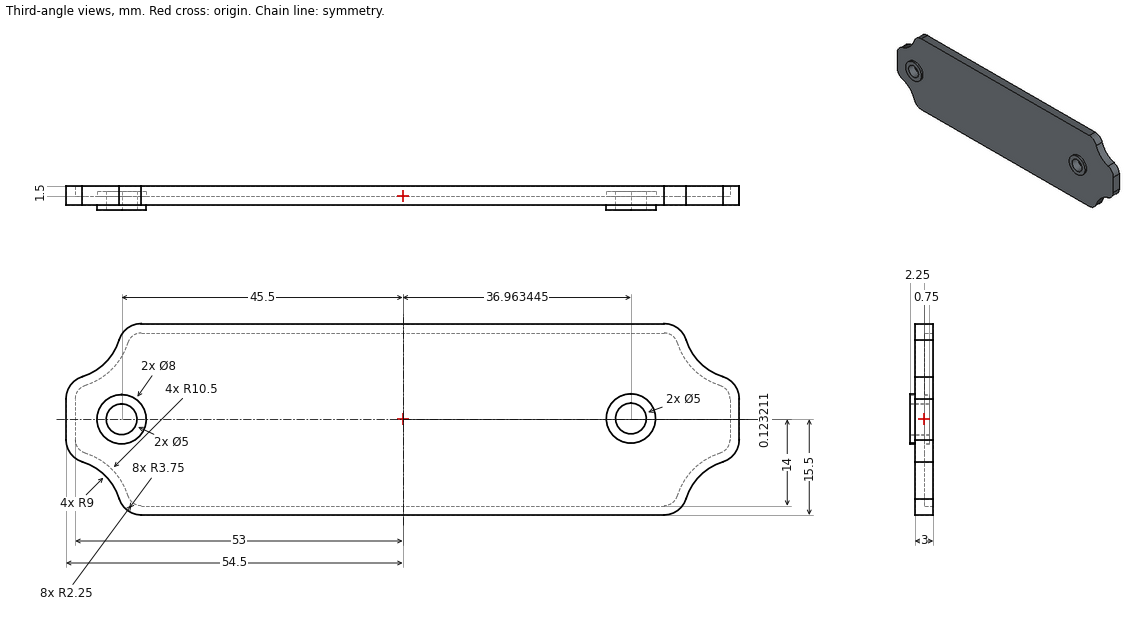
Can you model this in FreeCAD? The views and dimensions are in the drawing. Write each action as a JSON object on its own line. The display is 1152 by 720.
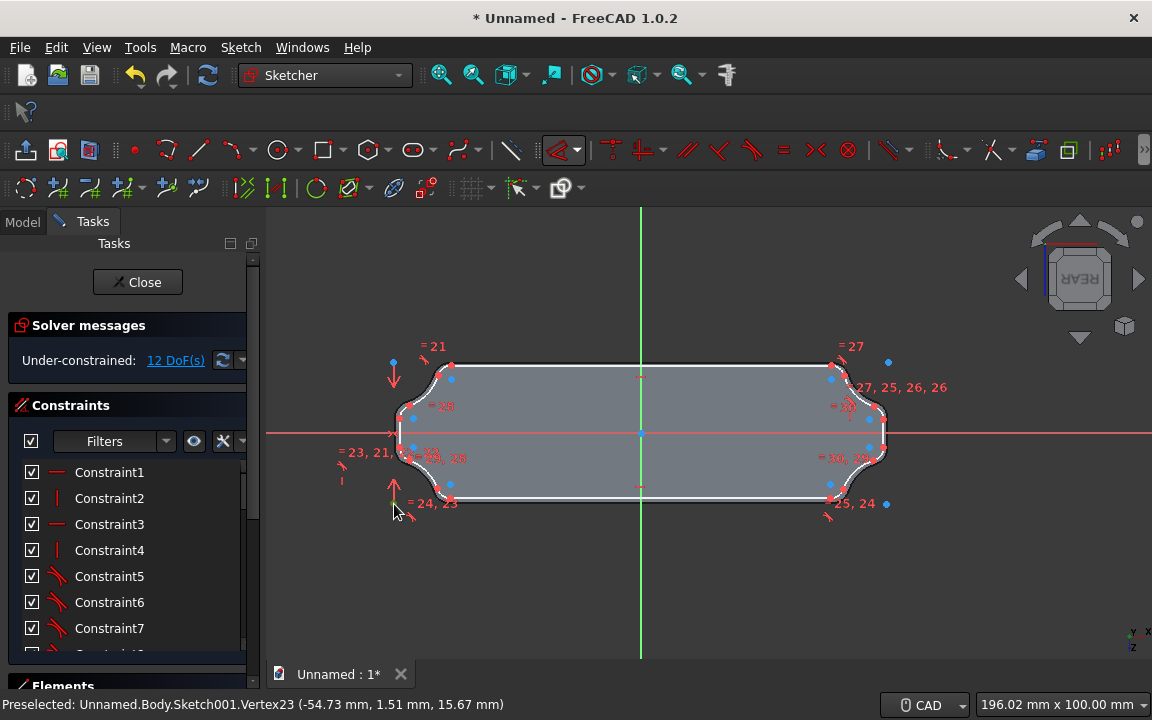
{"action": "left_click", "coordinate": [887, 505]}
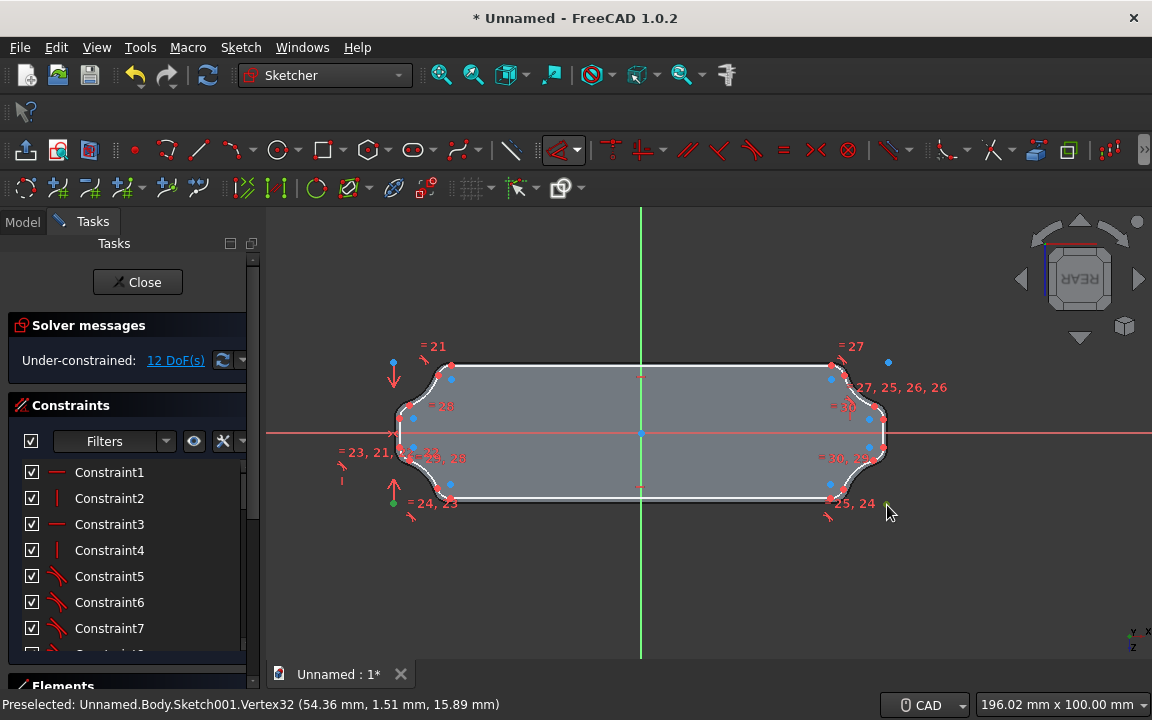
{"action": "left_click", "coordinate": [641, 603]}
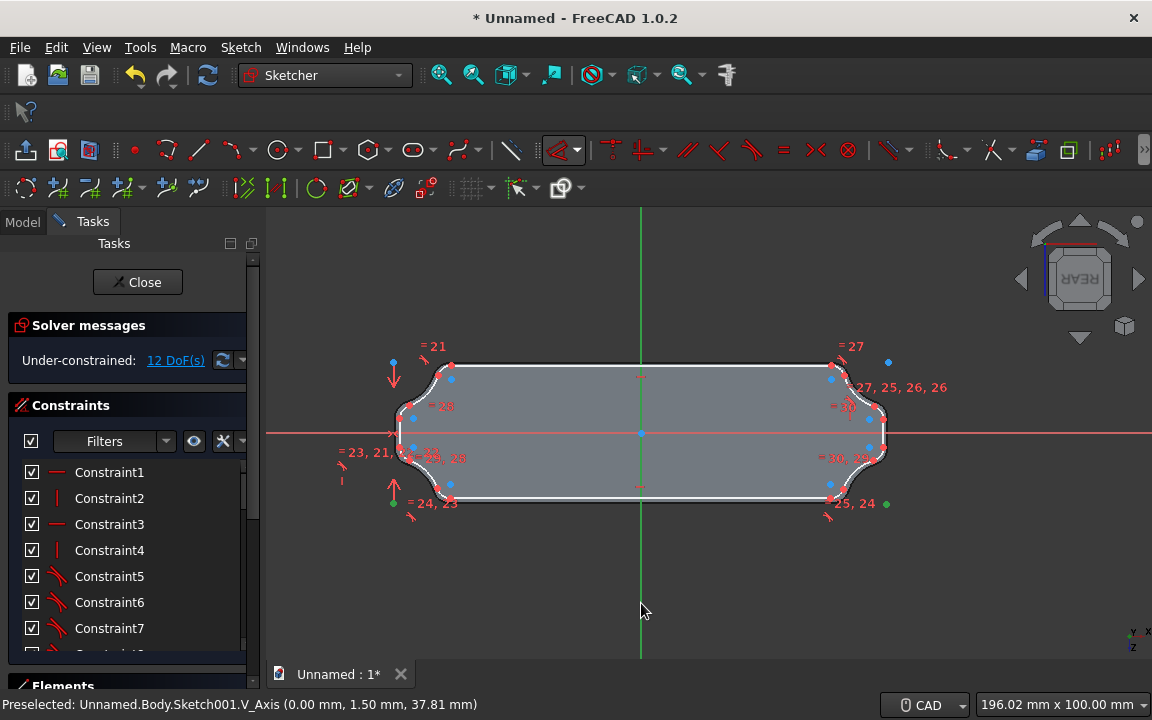
{"action": "left_click", "coordinate": [816, 150]}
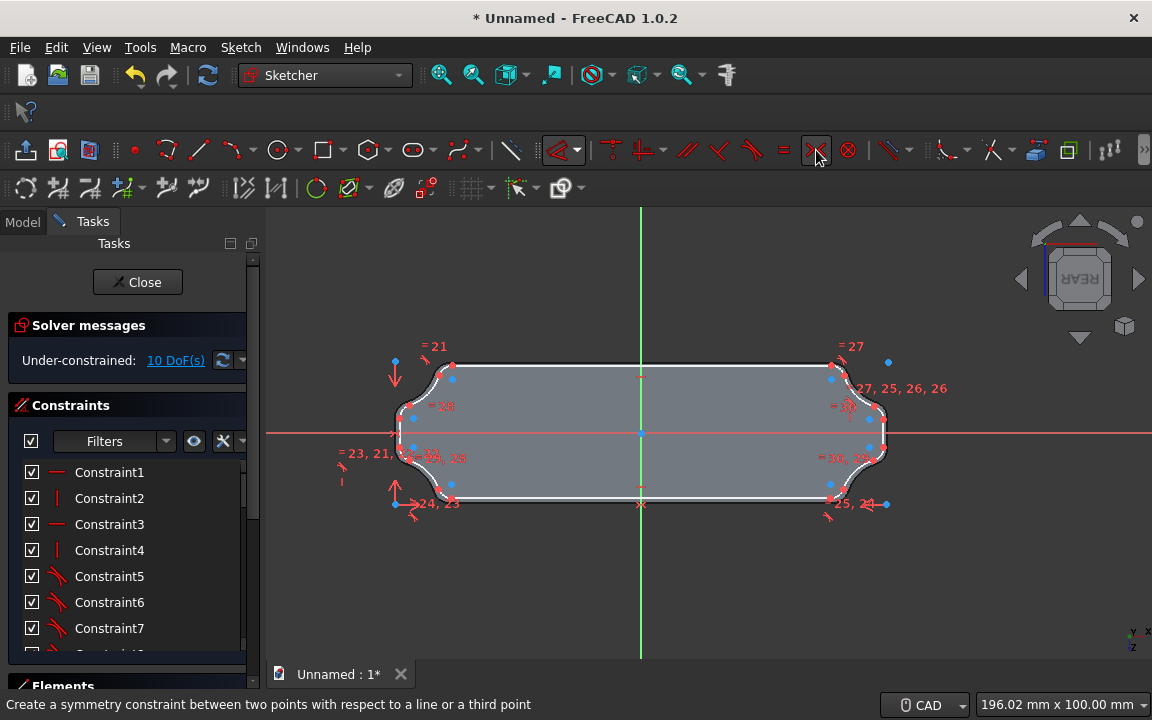
{"action": "left_click", "coordinate": [414, 418]}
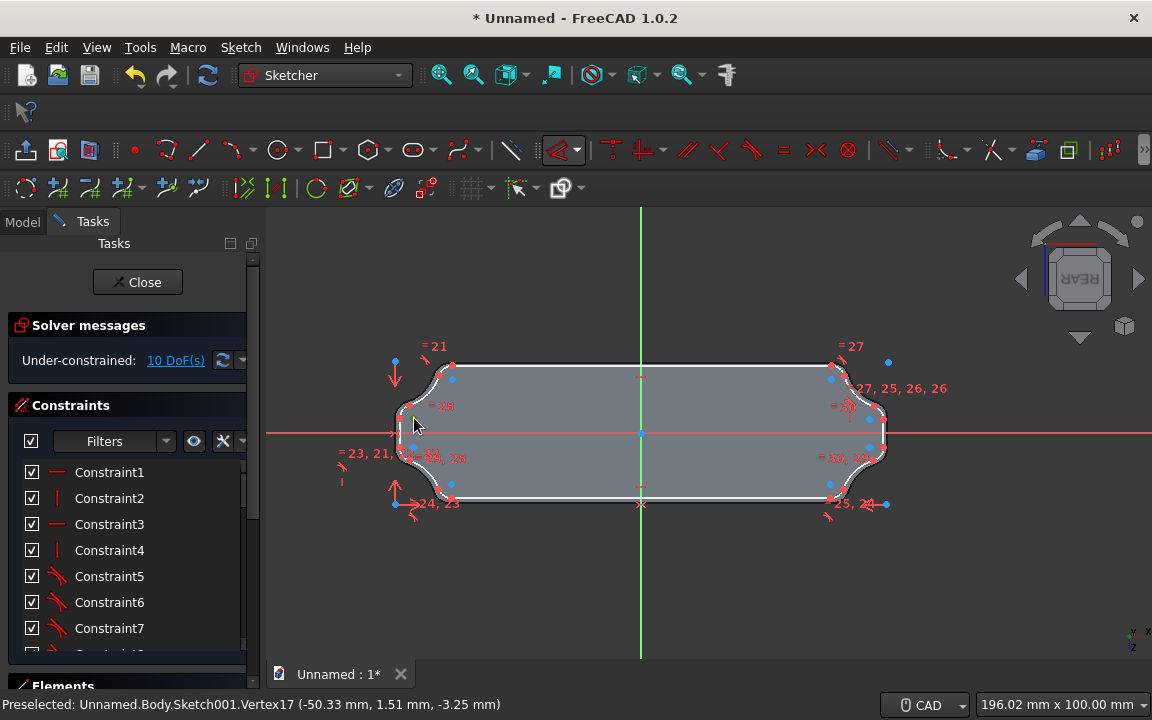
{"action": "left_click", "coordinate": [870, 420]}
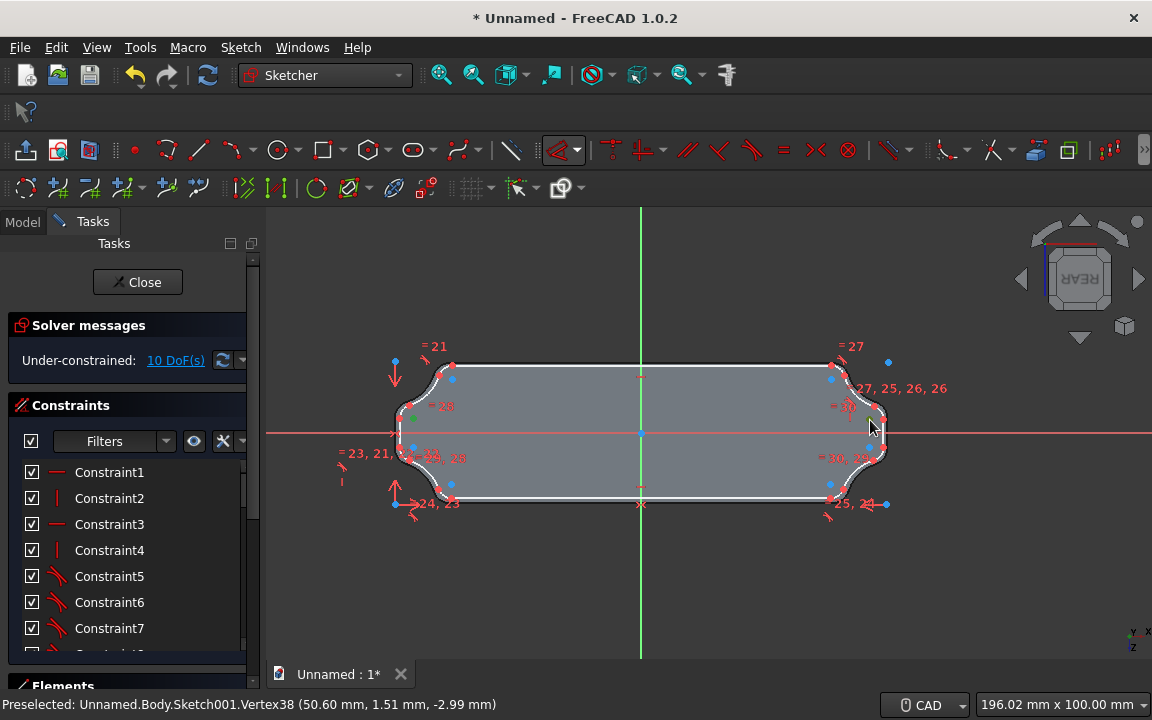
{"action": "left_click", "coordinate": [641, 603]}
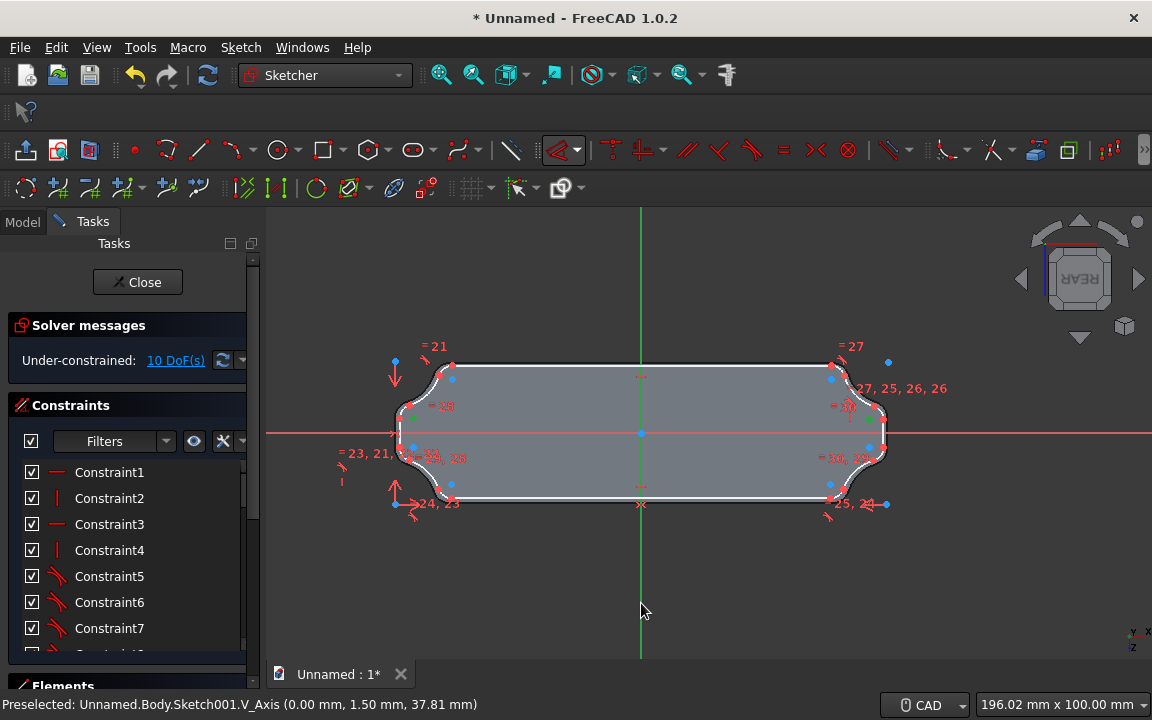
{"action": "left_click", "coordinate": [816, 150]}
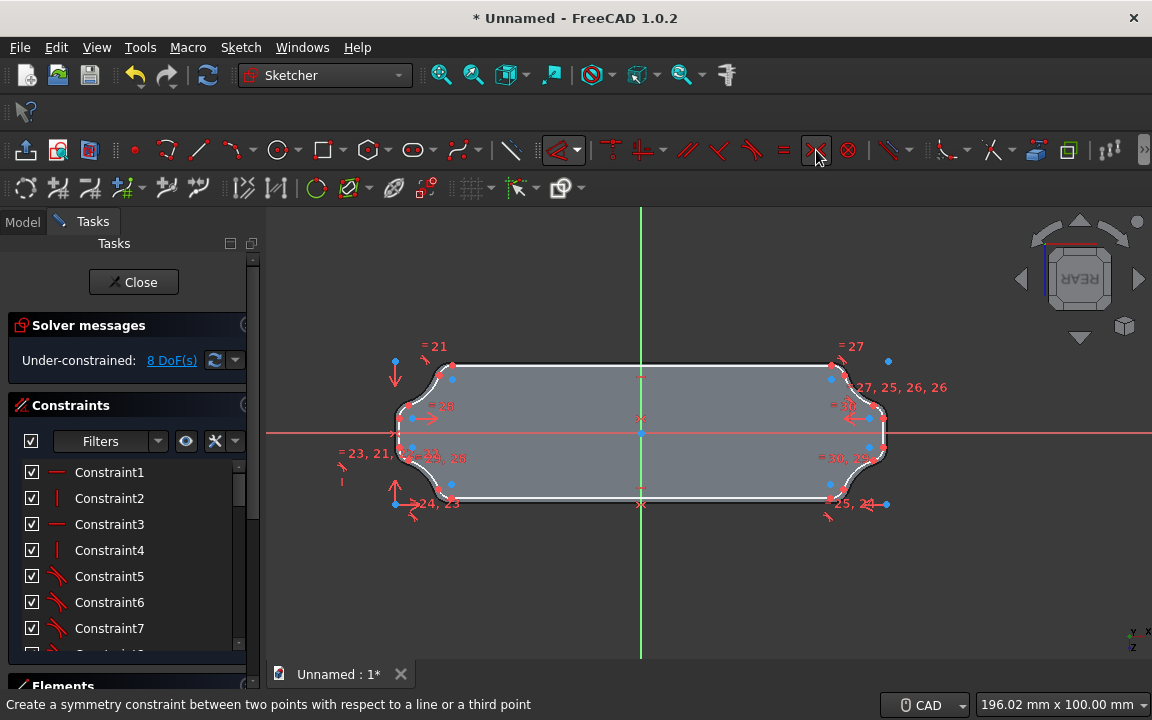
{"action": "left_click", "coordinate": [831, 485]}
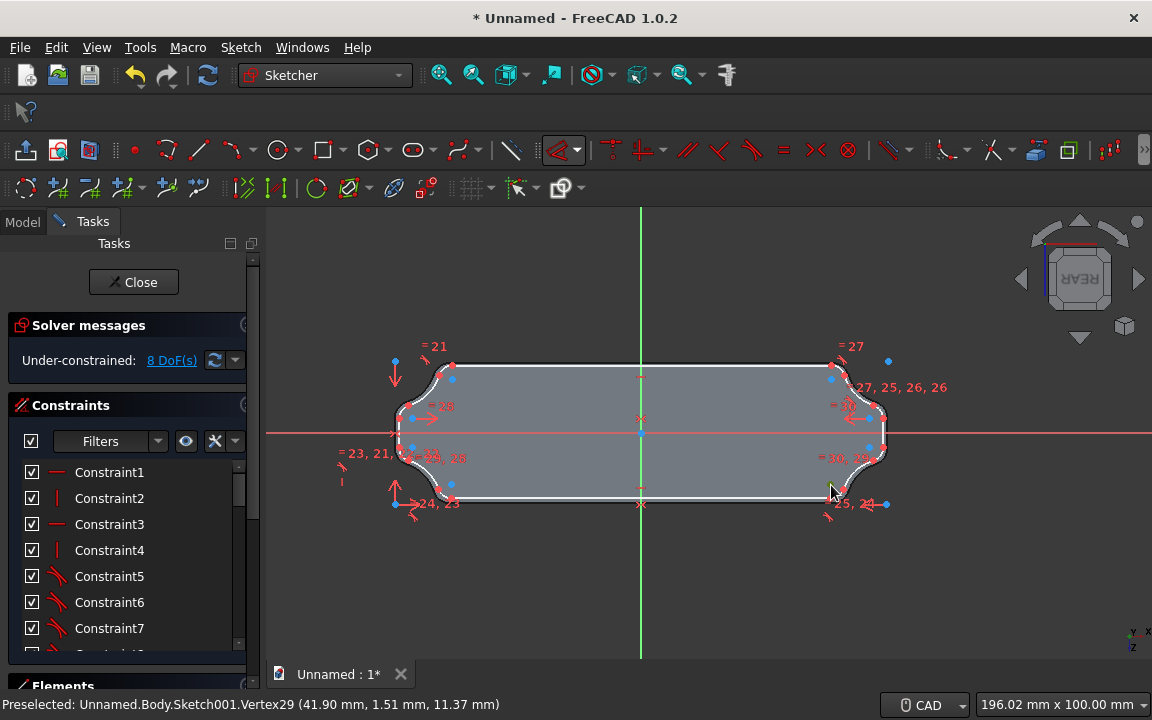
{"action": "left_click", "coordinate": [831, 379]}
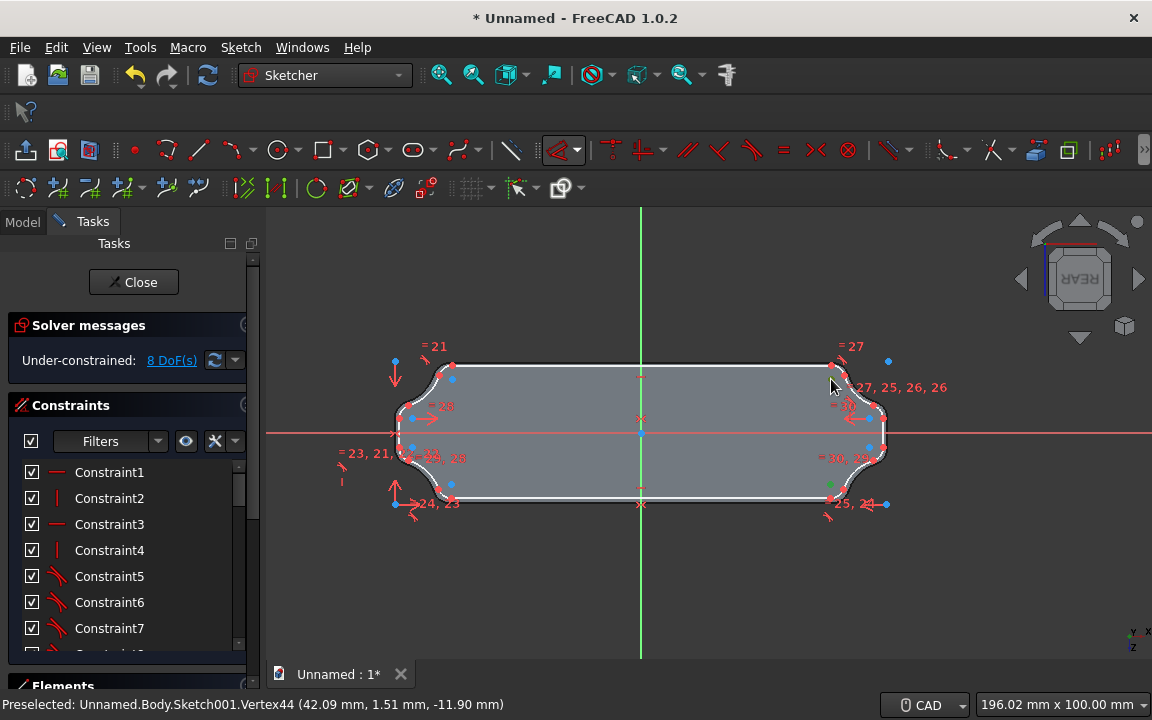
{"action": "left_click", "coordinate": [344, 433]}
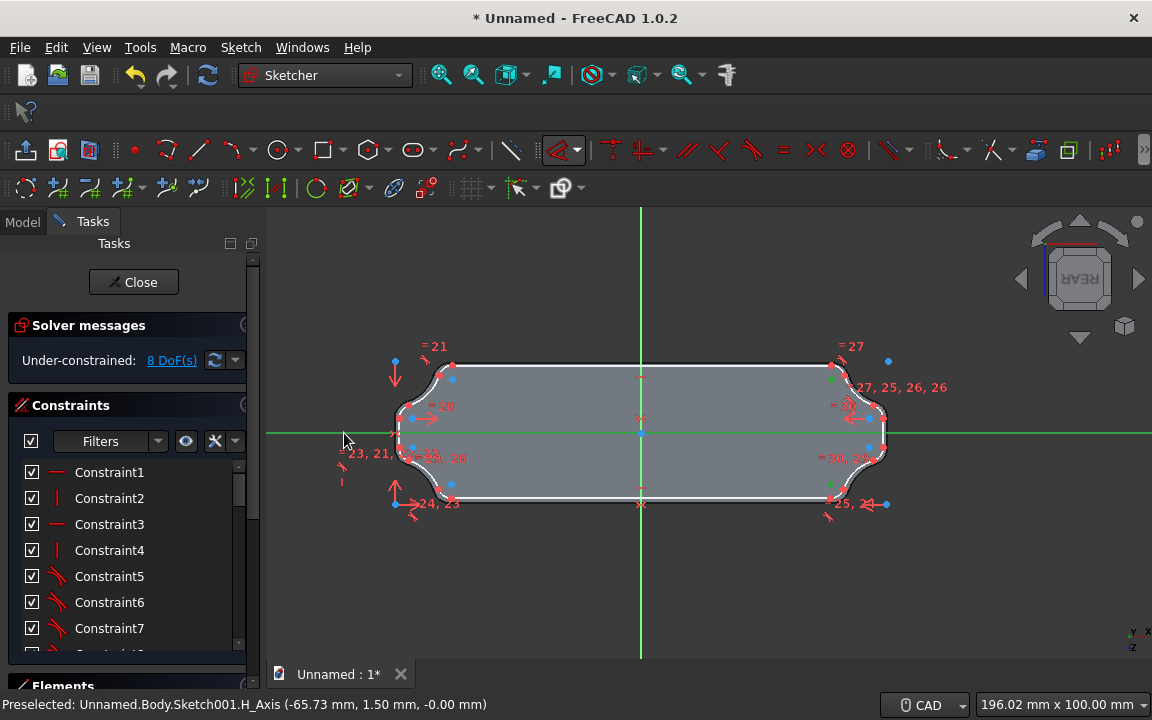
{"action": "left_click", "coordinate": [816, 150]}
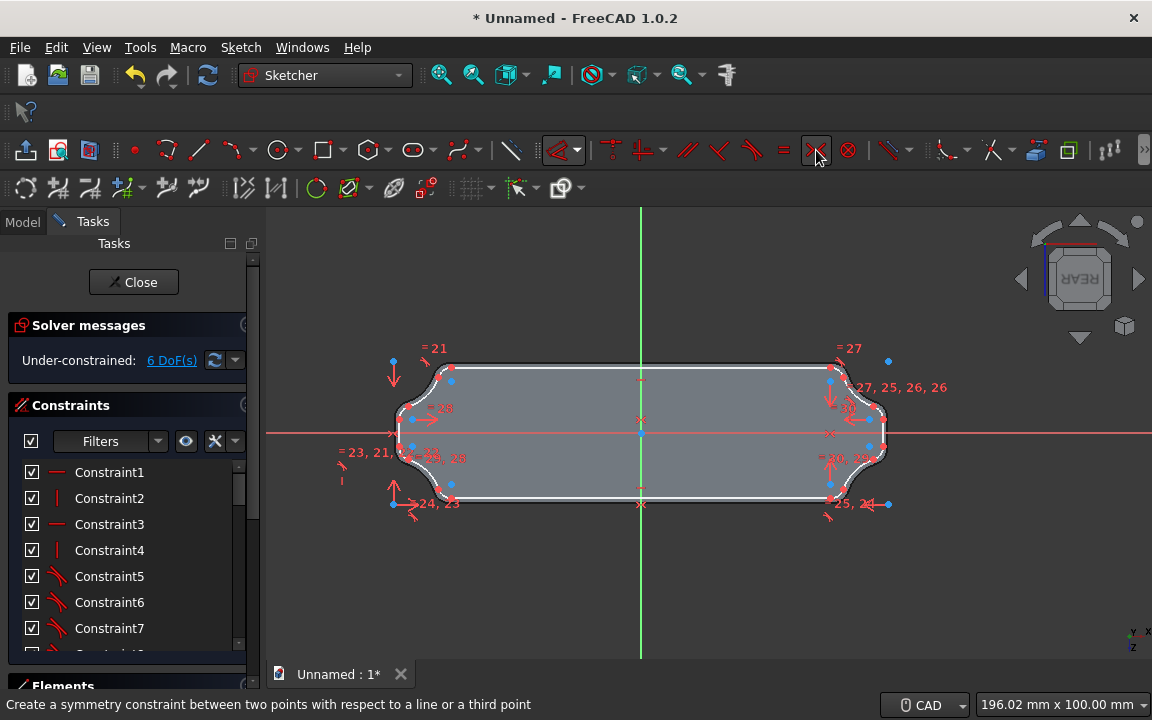
{"action": "scroll", "coordinate": [444, 370], "scroll_direction": "up", "scroll_amount": 7}